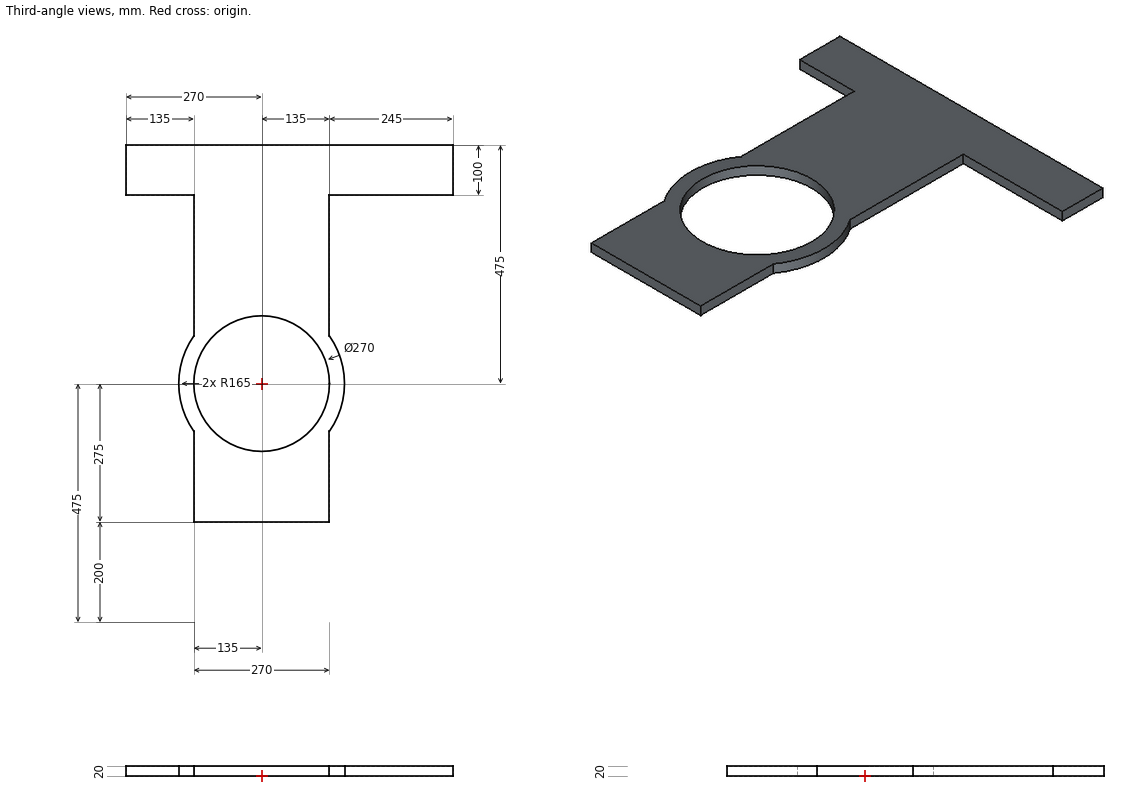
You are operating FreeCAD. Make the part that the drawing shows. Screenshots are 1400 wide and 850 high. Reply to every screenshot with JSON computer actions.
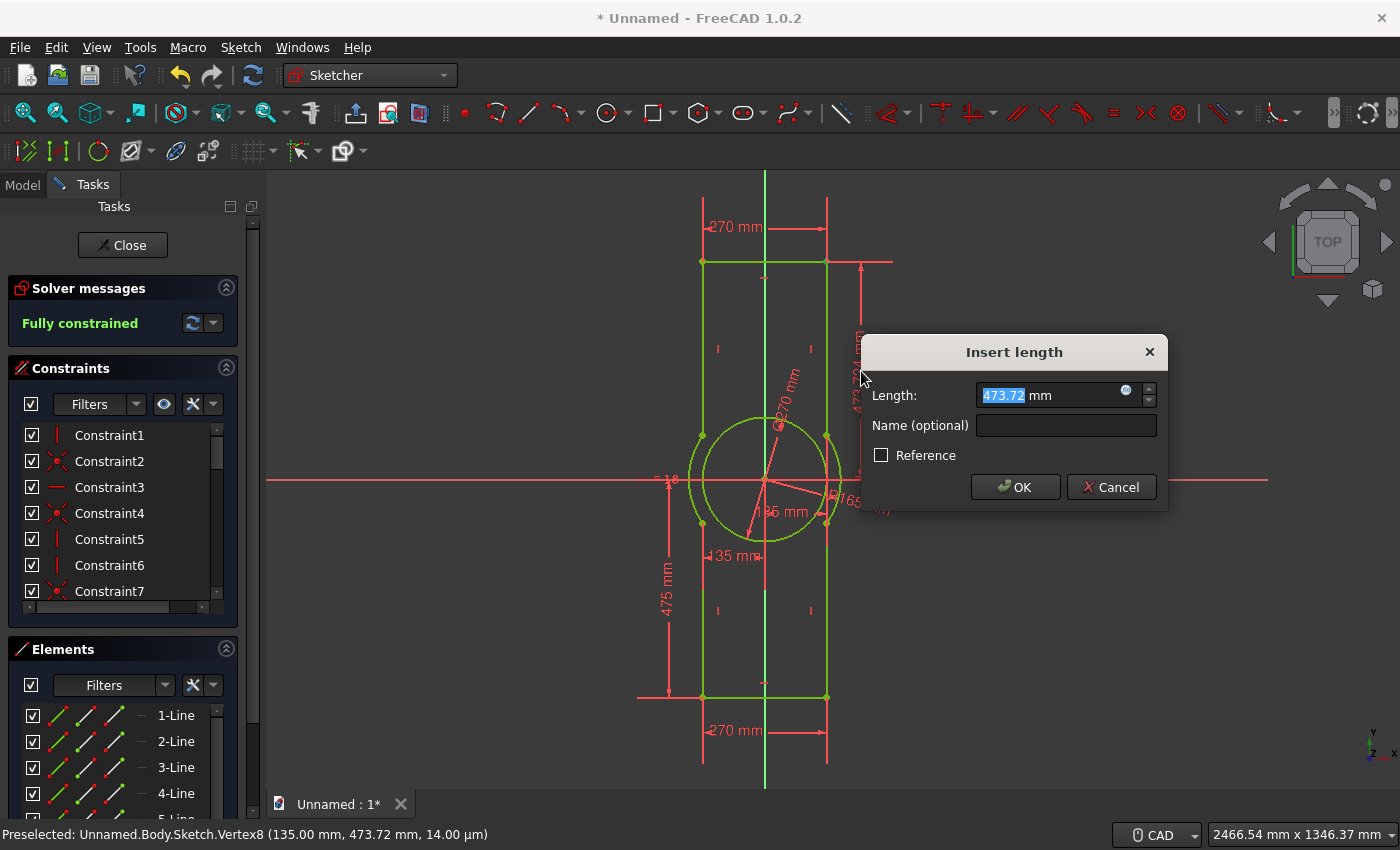
{"action": "type", "text": "475"}
{"action": "key", "text": "Return"}
{"action": "key", "text": "Escape"}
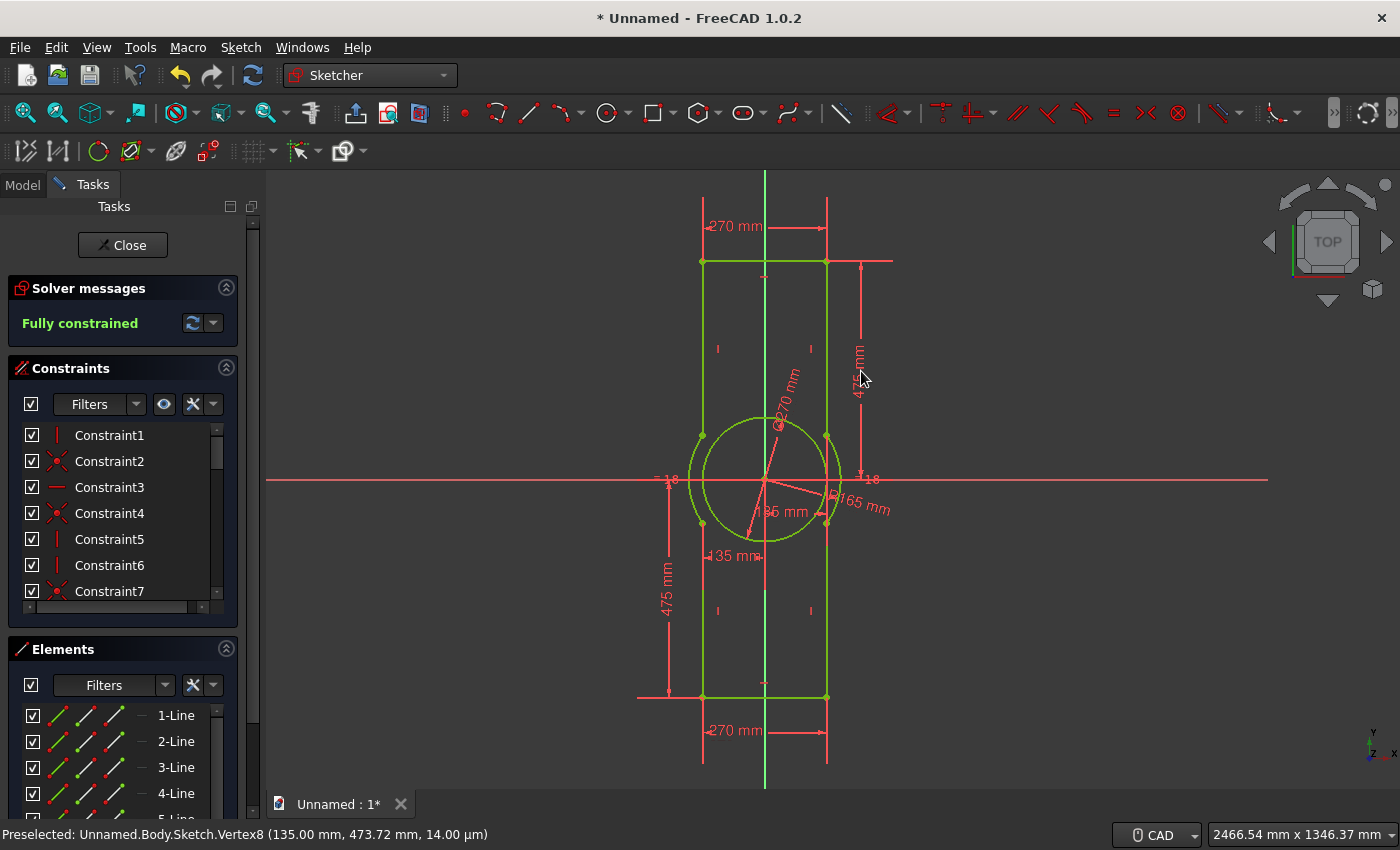
{"action": "left_click", "coordinate": [123, 245]}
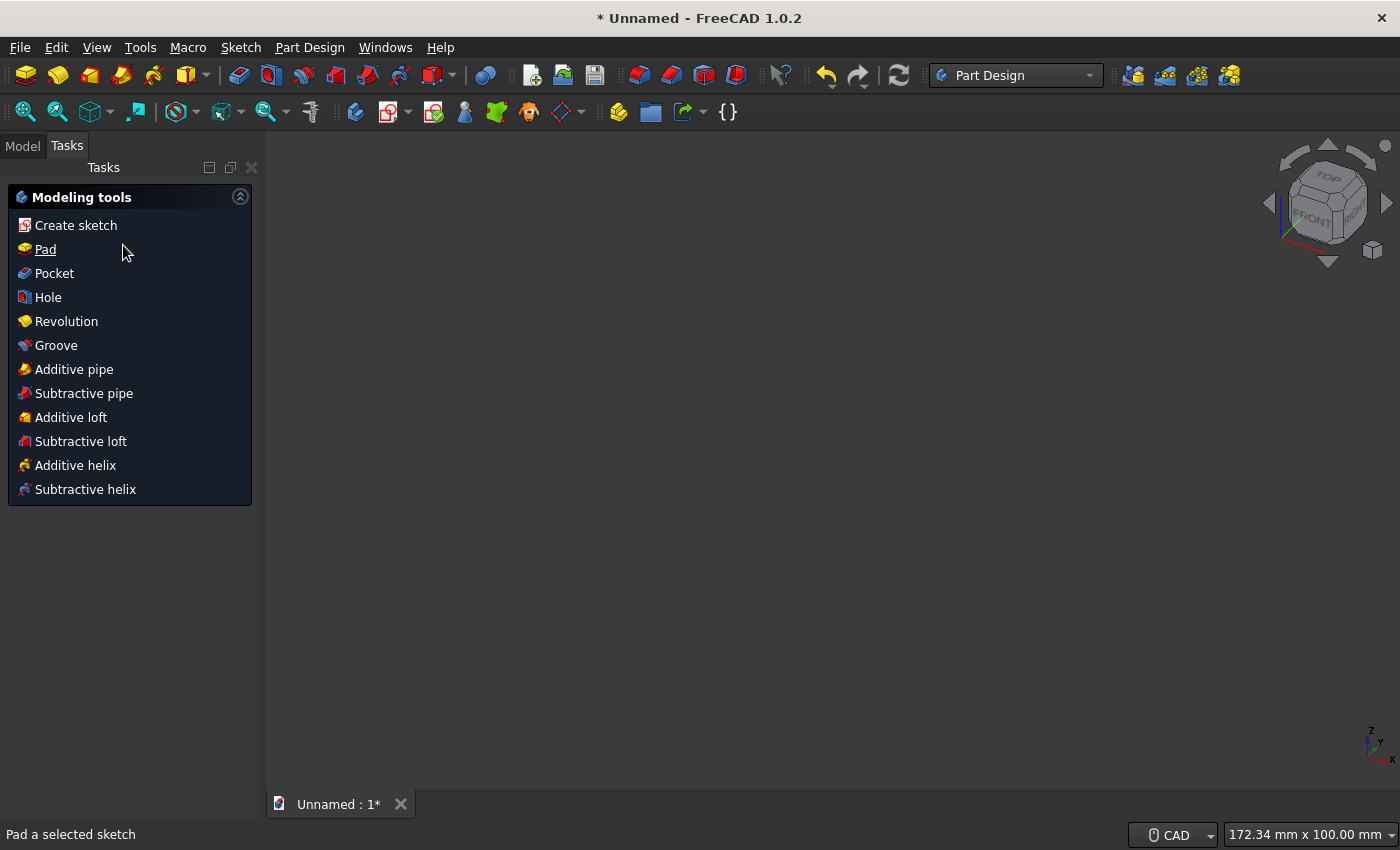
{"action": "left_click", "coordinate": [26, 76]}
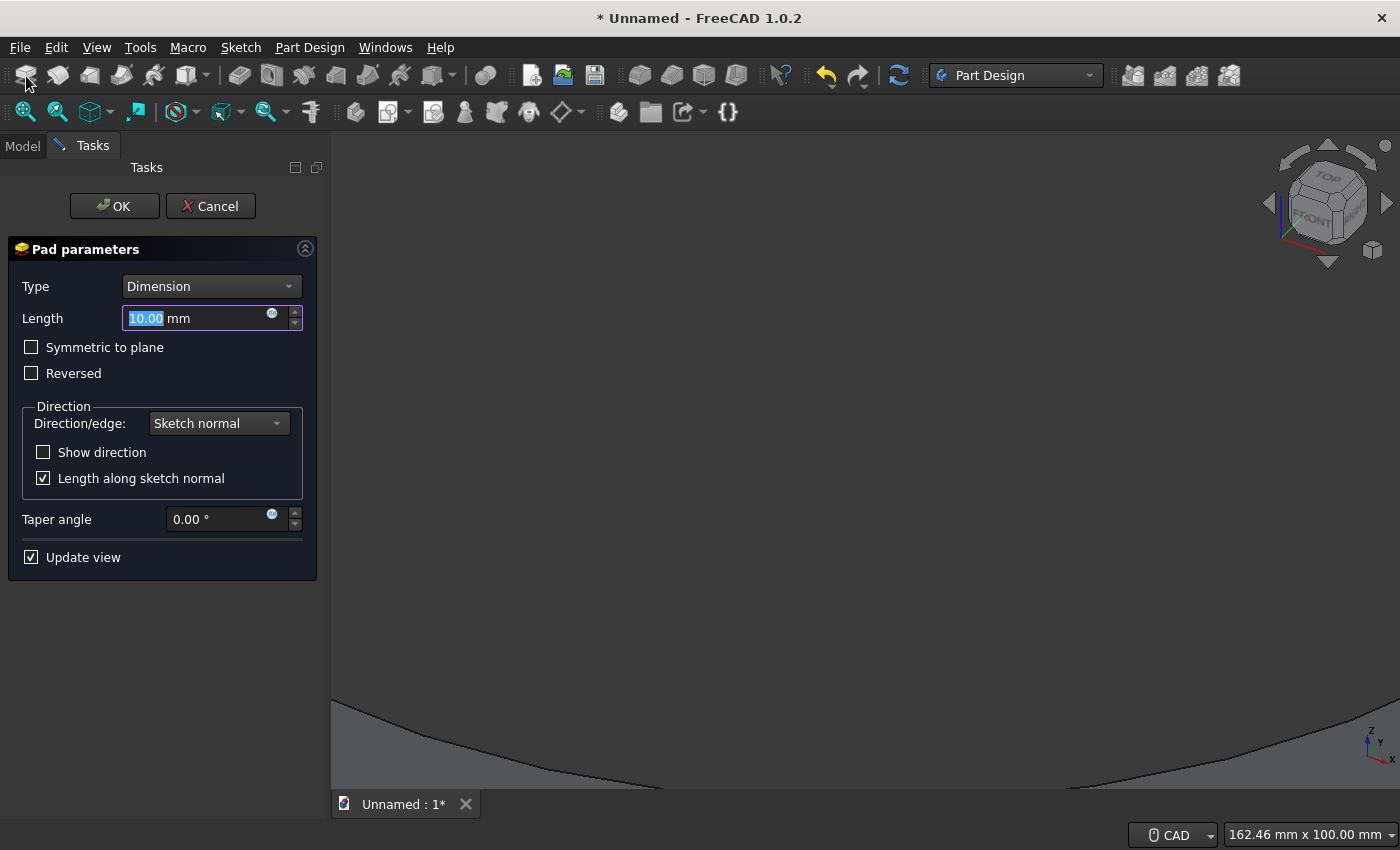
{"action": "type", "text": "20"}
{"action": "key", "text": "Tab"}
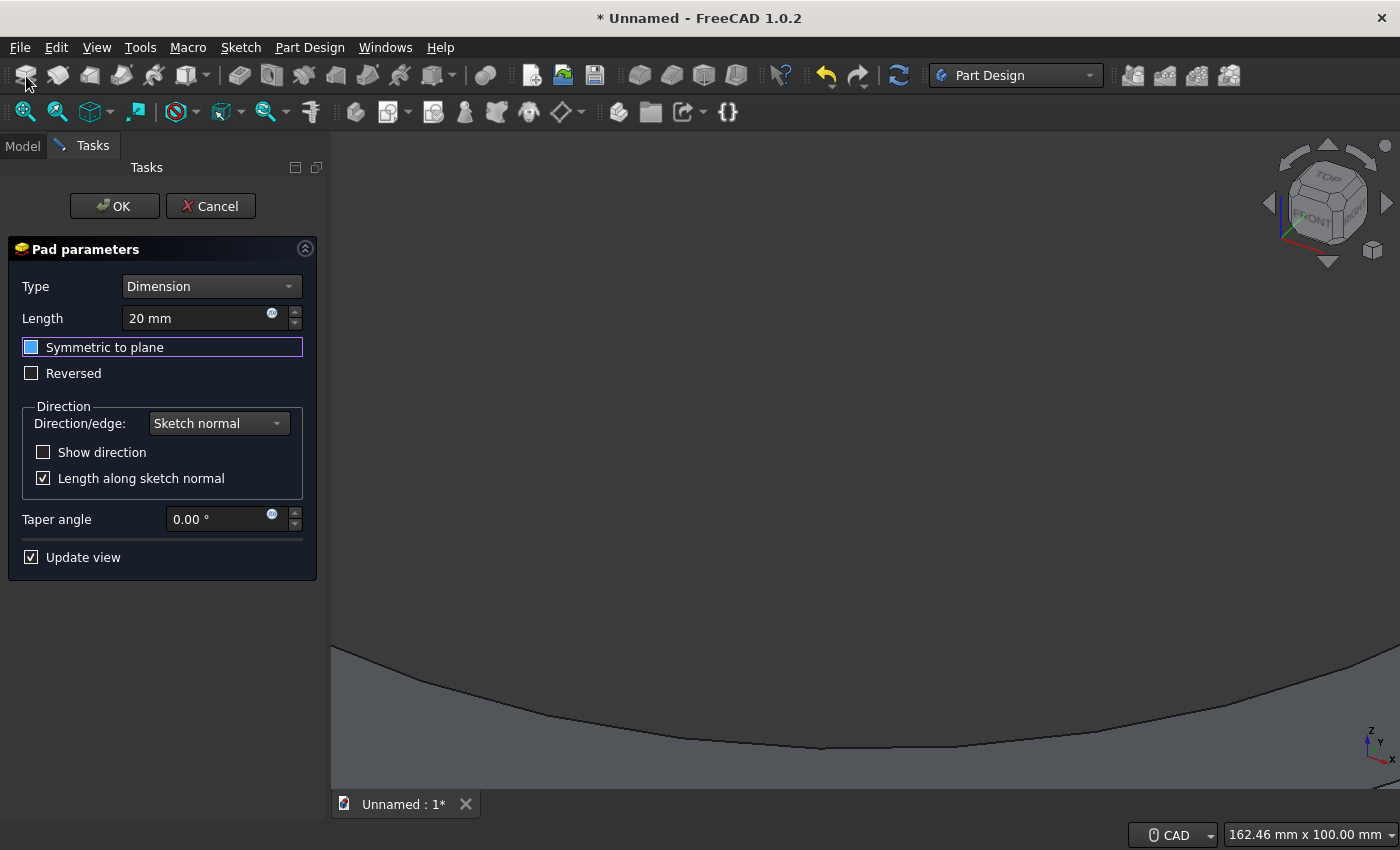
{"action": "left_click", "coordinate": [115, 206]}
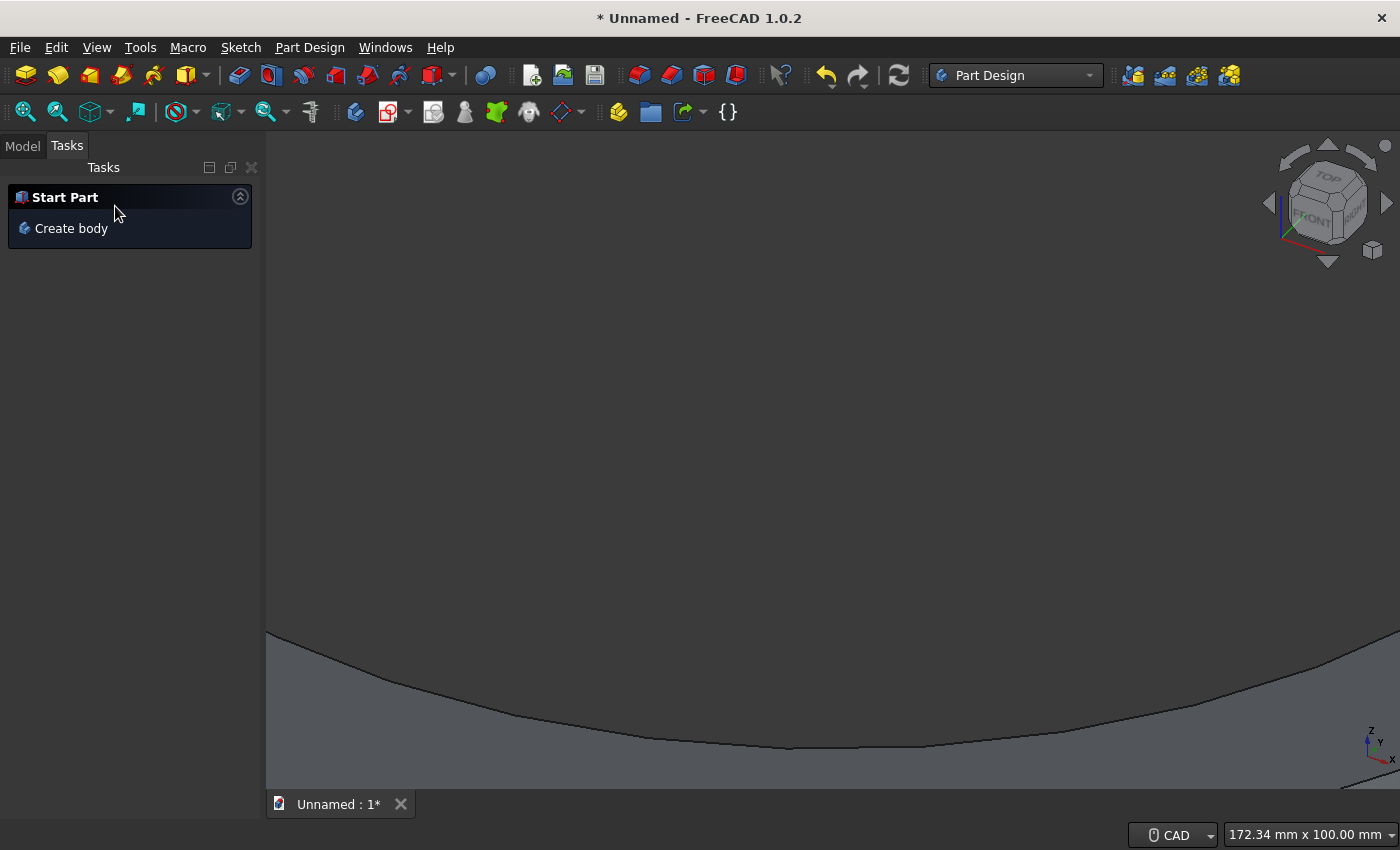
{"action": "key", "text": "v f"}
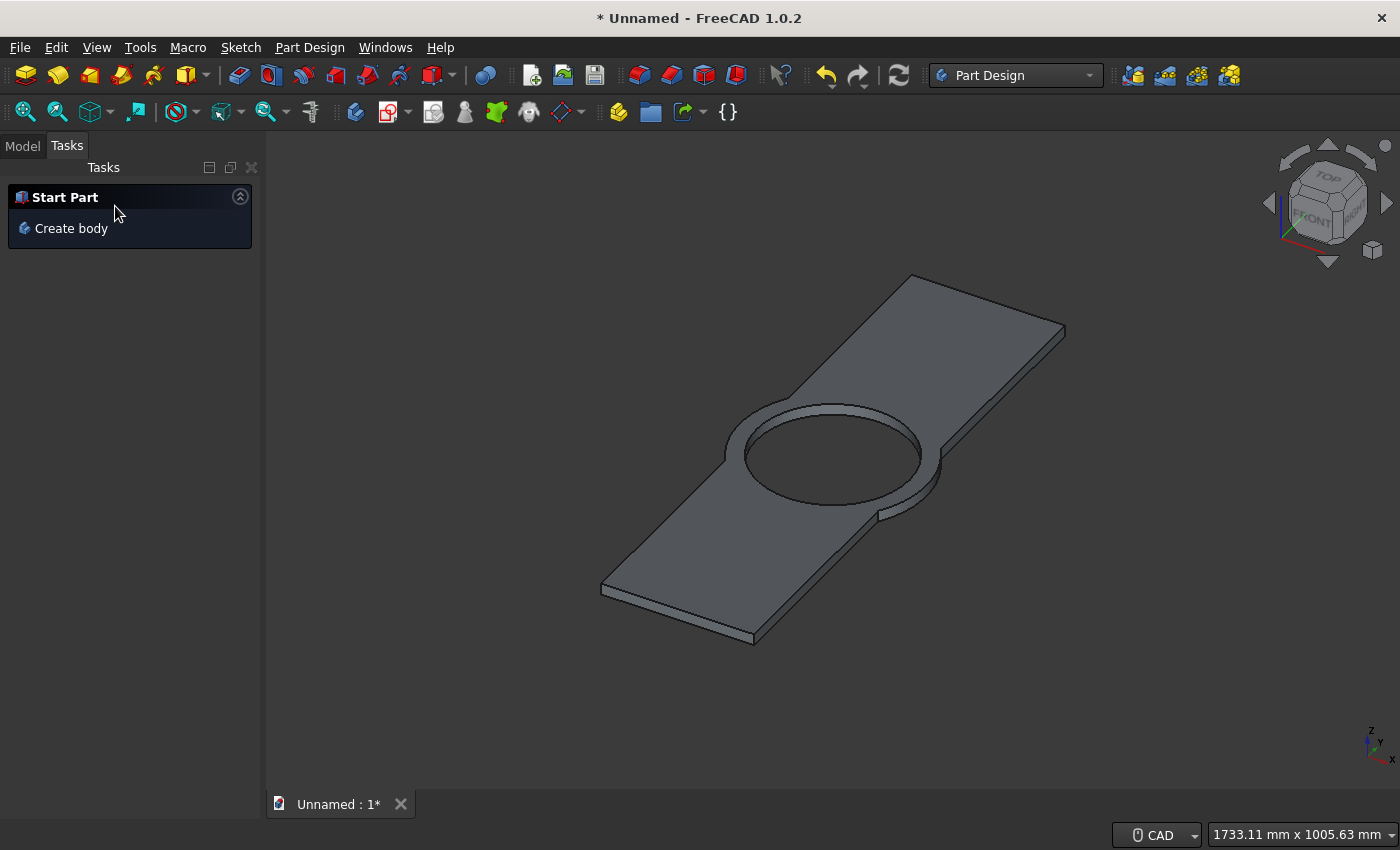
{"action": "left_click", "coordinate": [922, 365]}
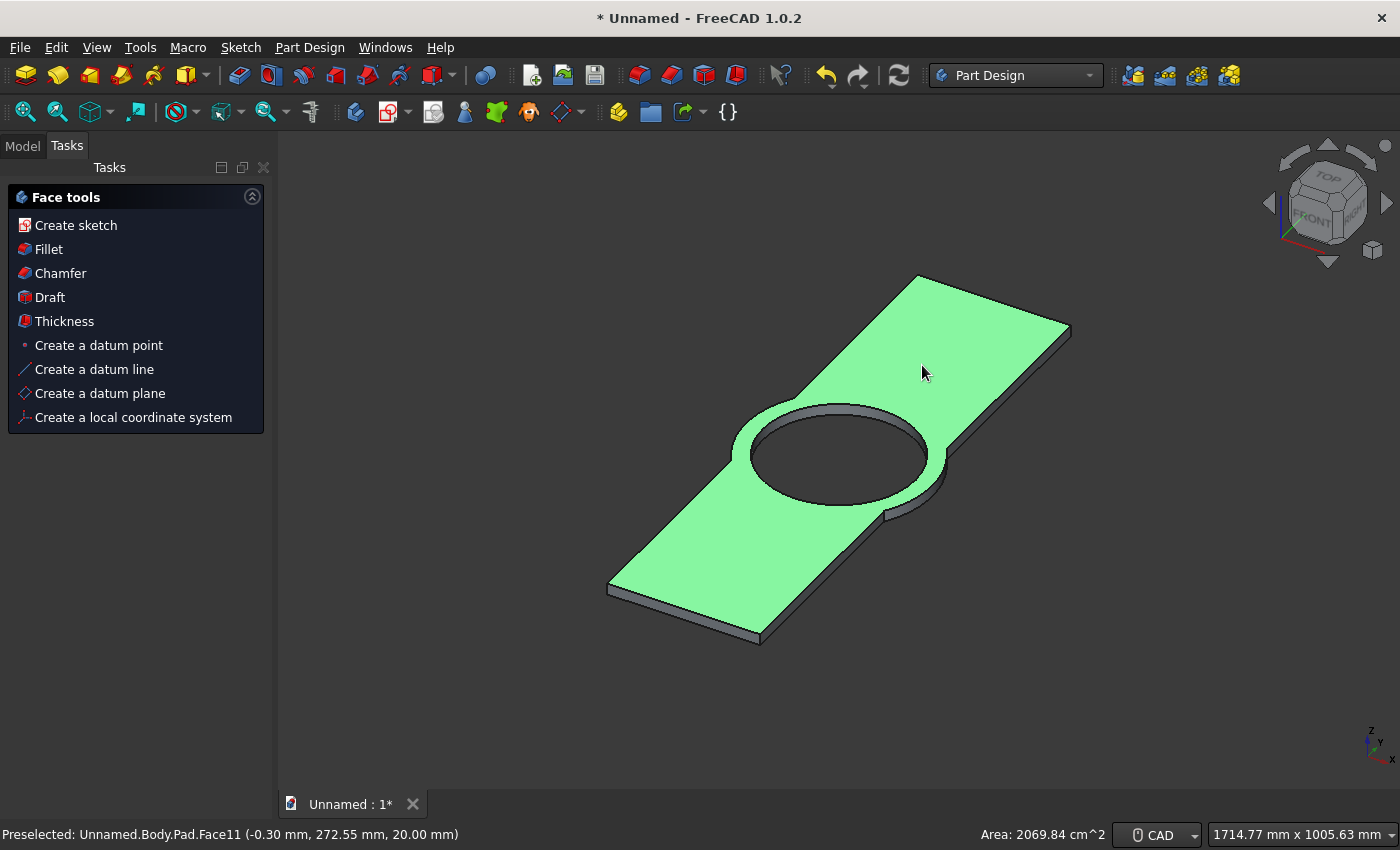
{"action": "left_click", "coordinate": [388, 112]}